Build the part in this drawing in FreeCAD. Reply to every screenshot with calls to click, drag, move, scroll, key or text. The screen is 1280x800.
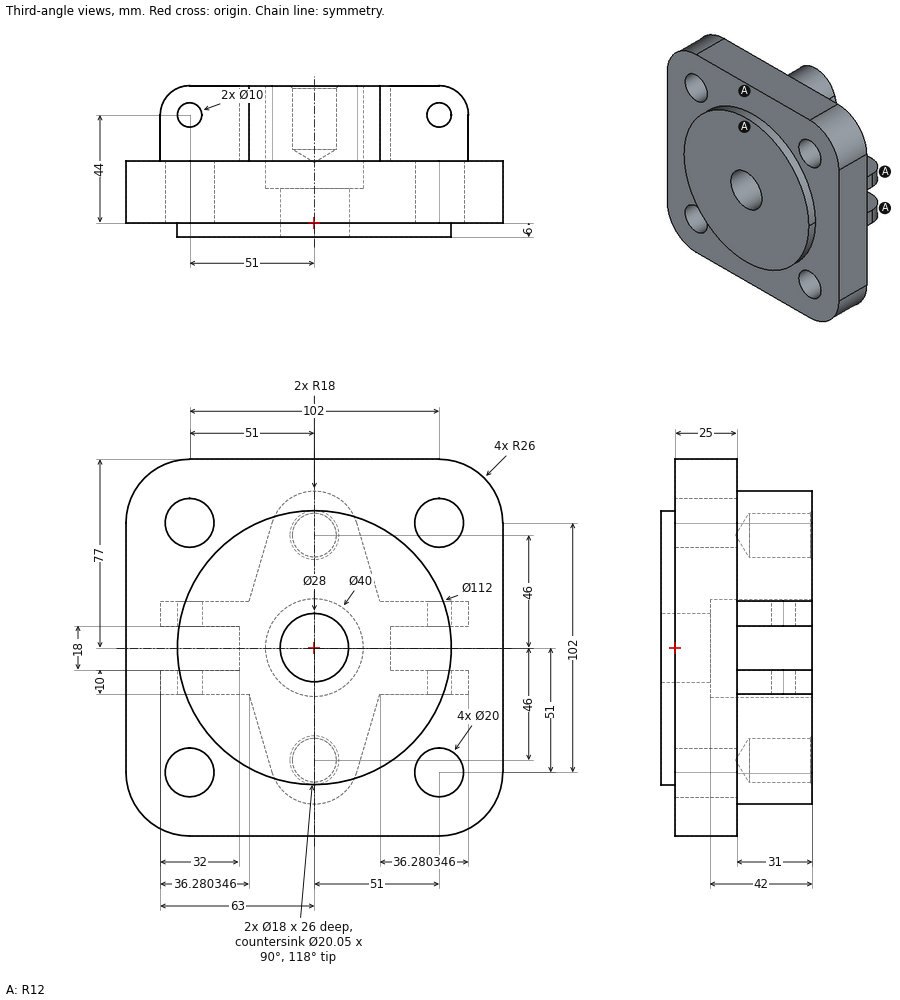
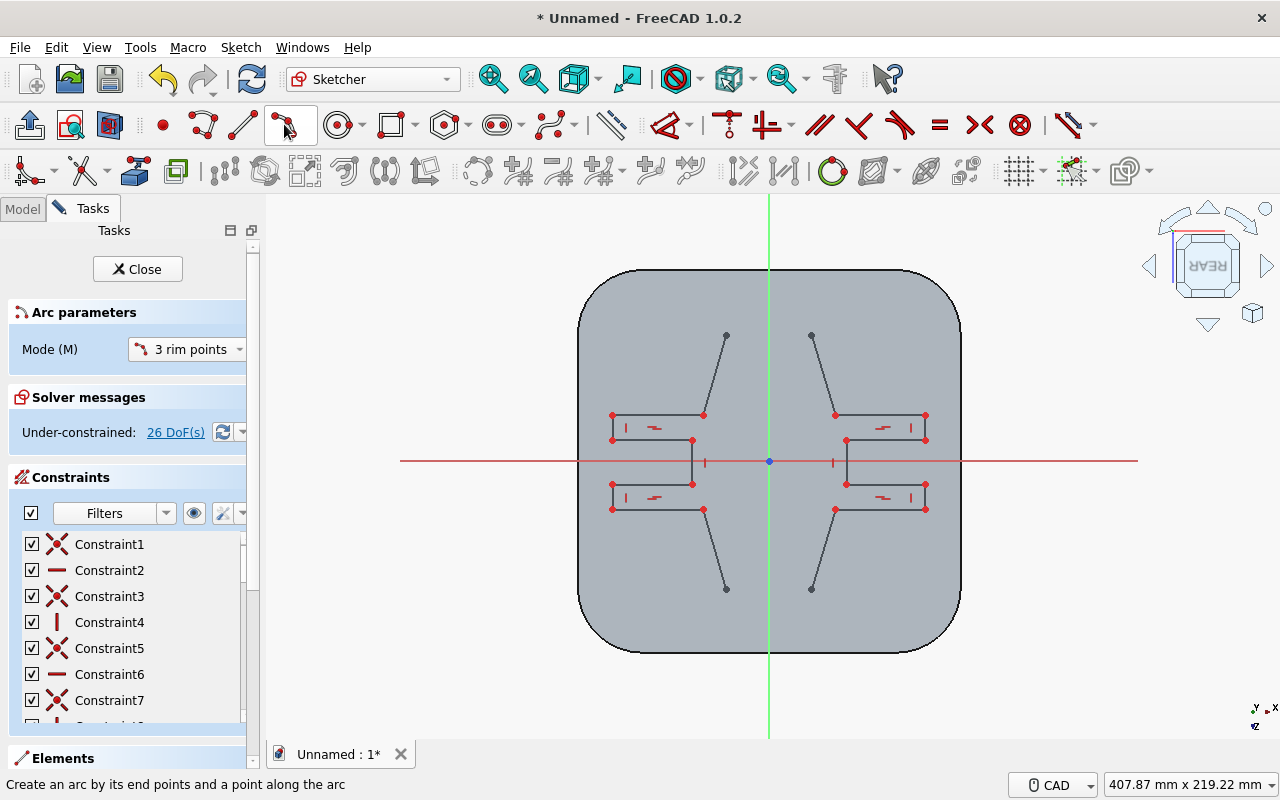
click(726, 590)
click(812, 590)
click(747, 615)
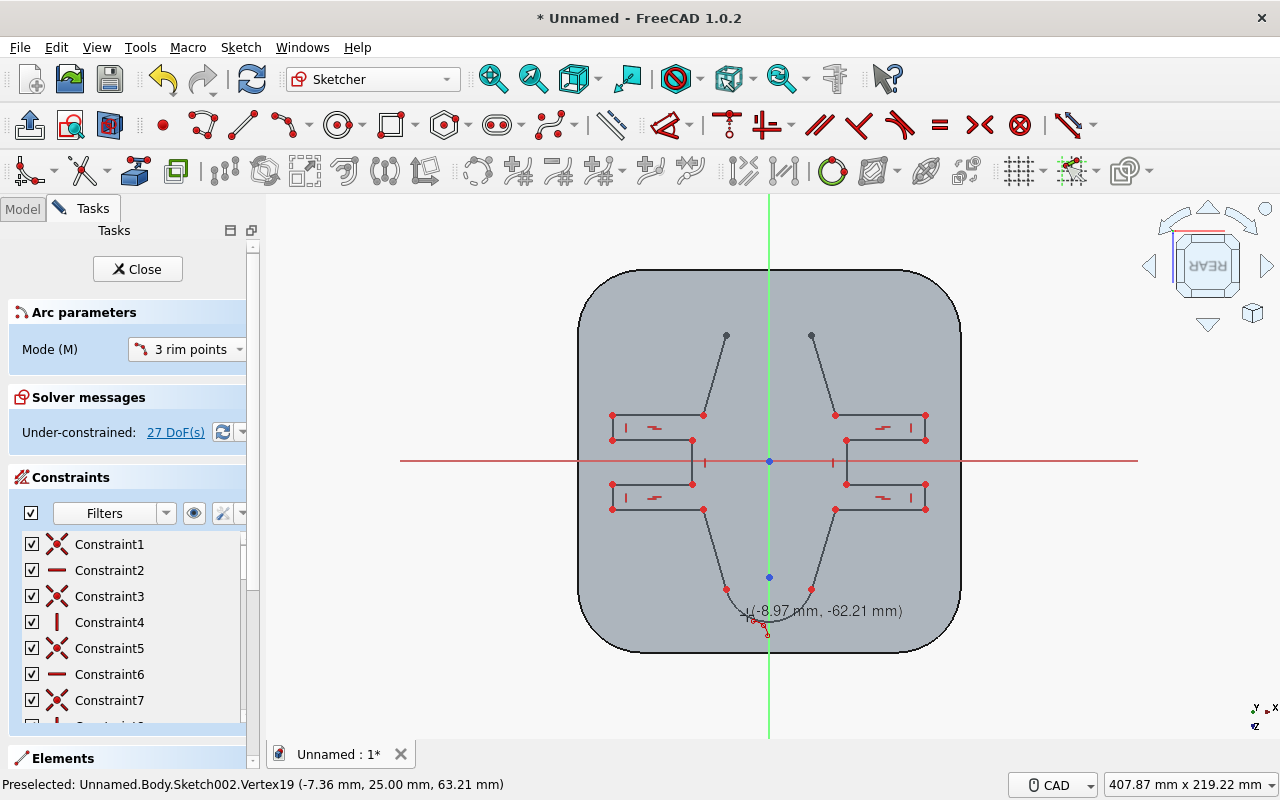
click(812, 335)
click(726, 335)
click(791, 308)
key(Escape)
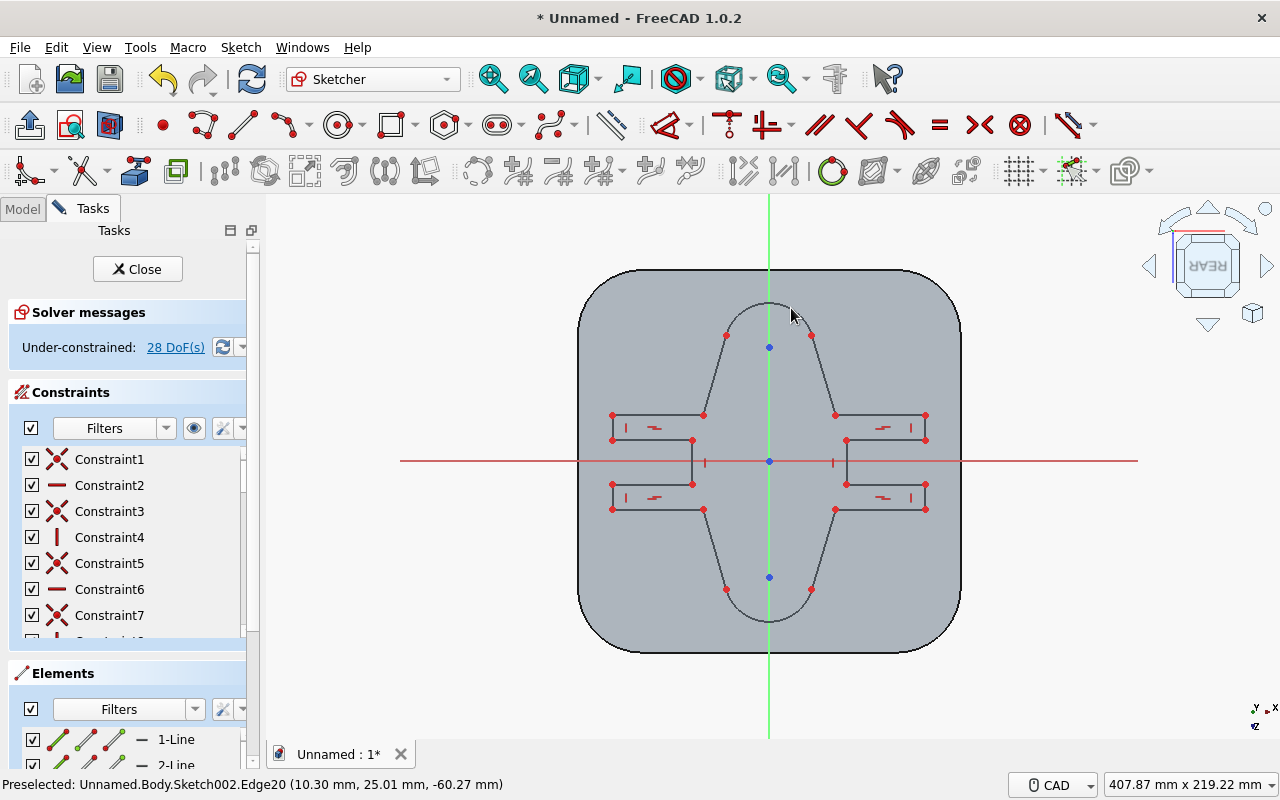
click(719, 359)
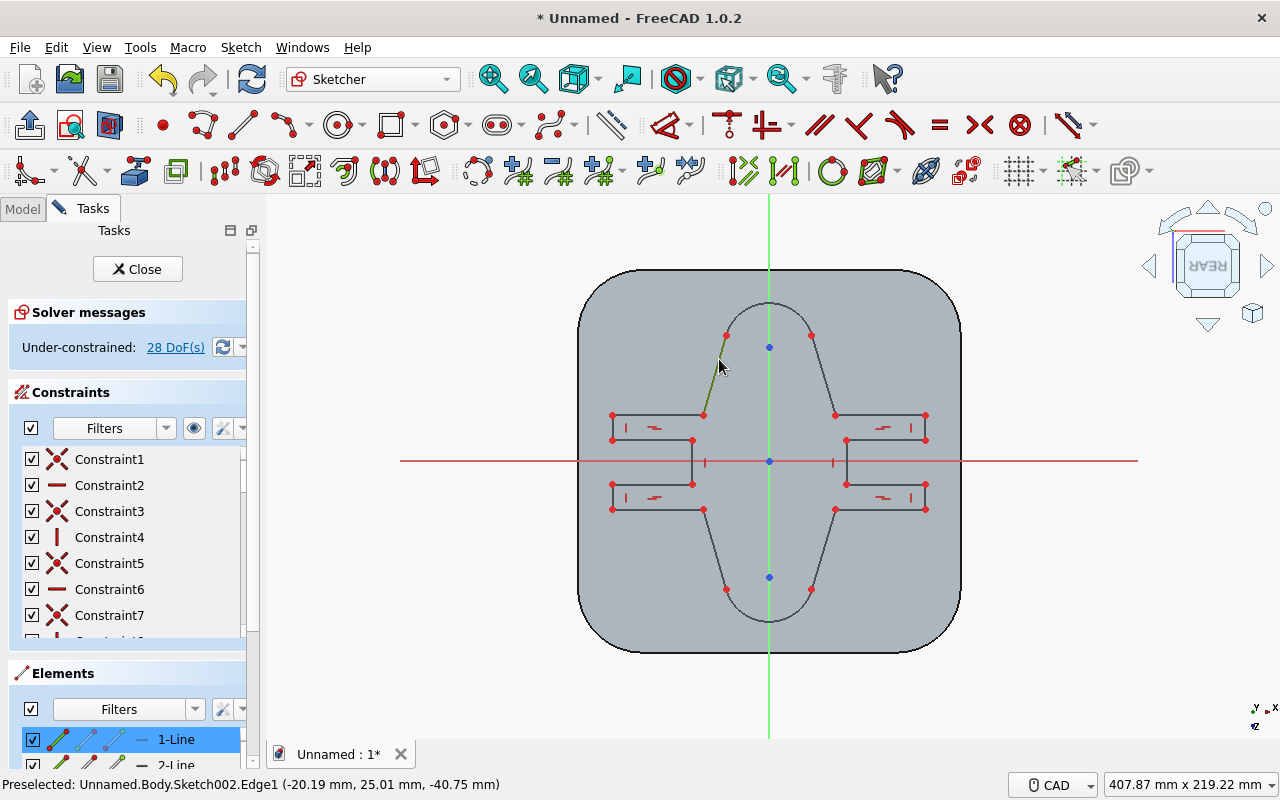
click(791, 309)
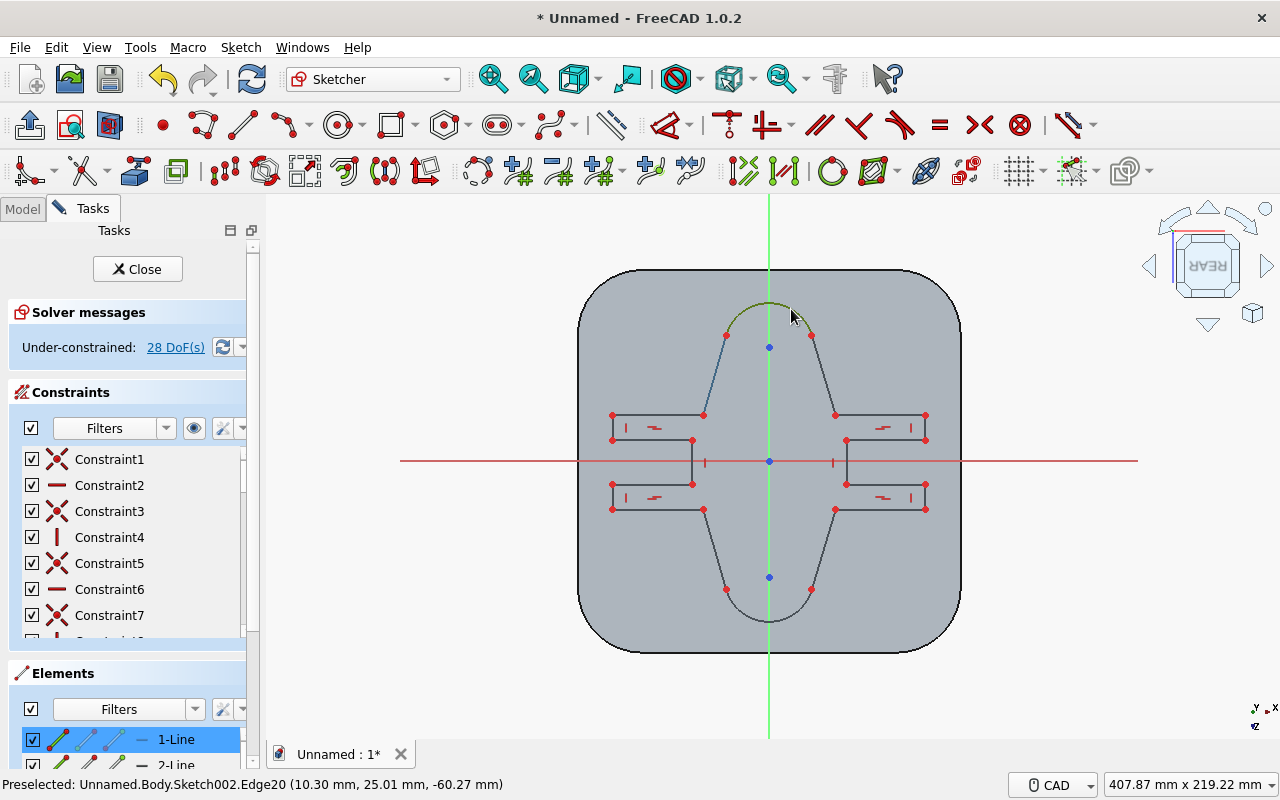
key(t)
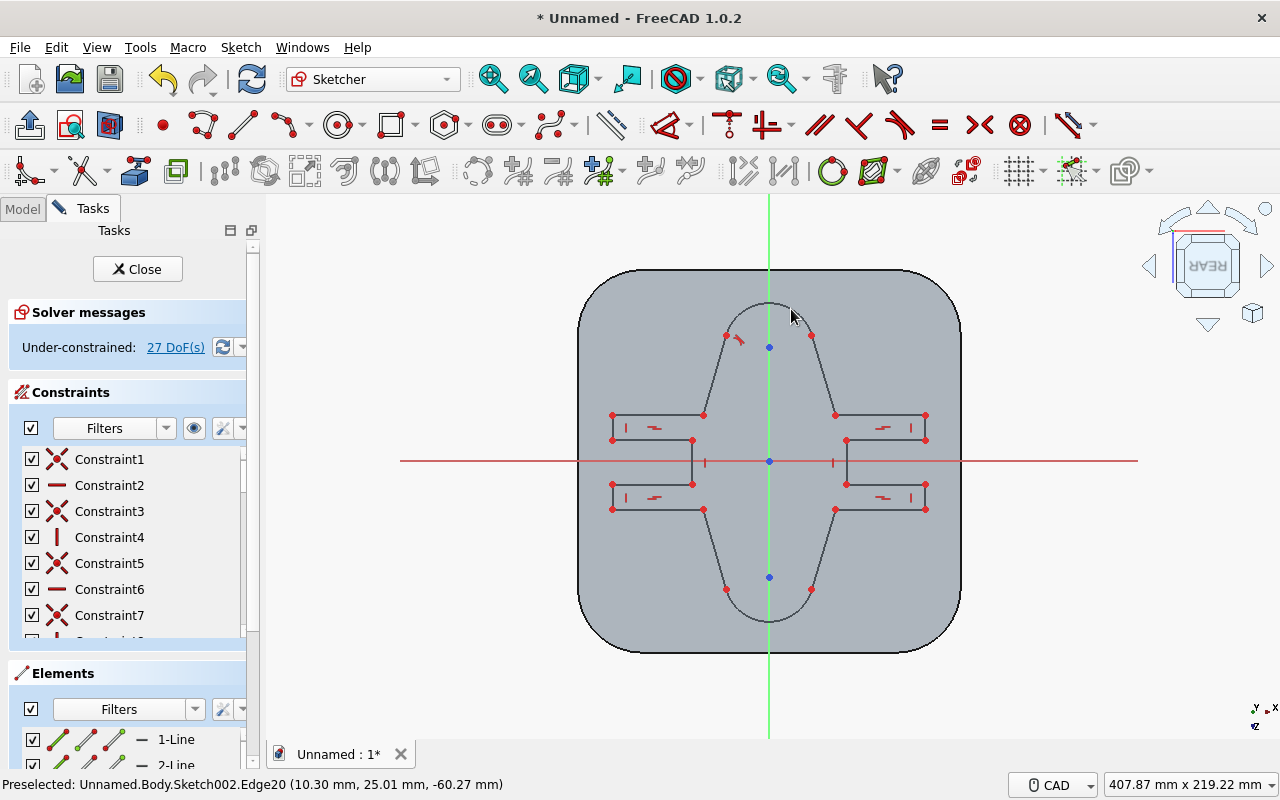
click(710, 534)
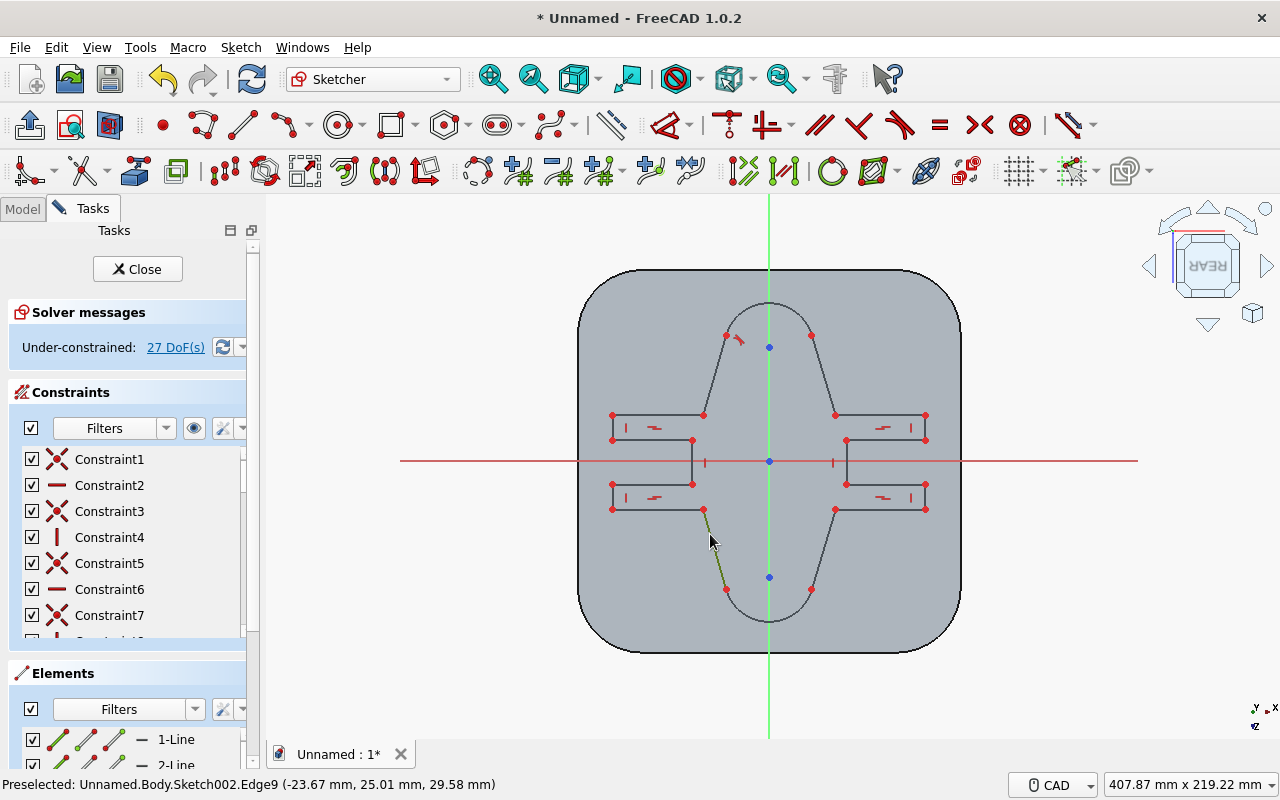
click(747, 616)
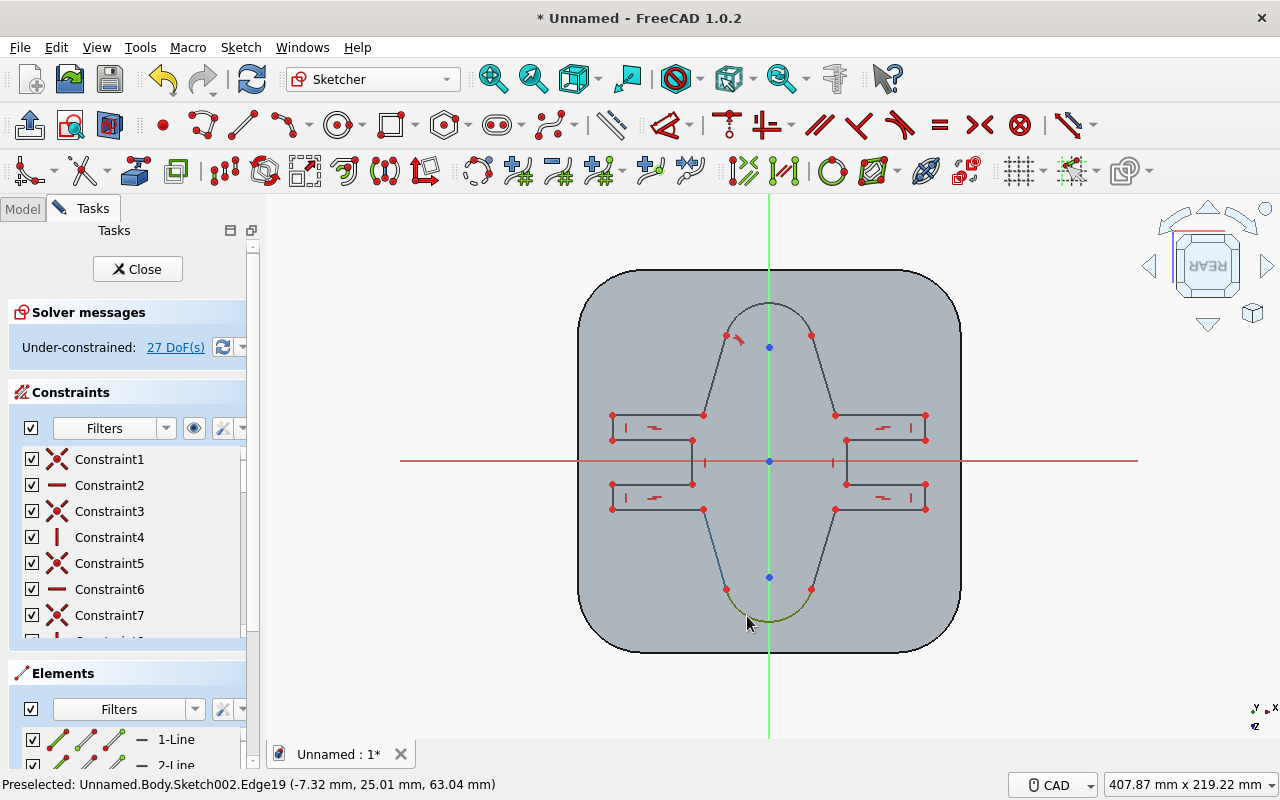
key(t)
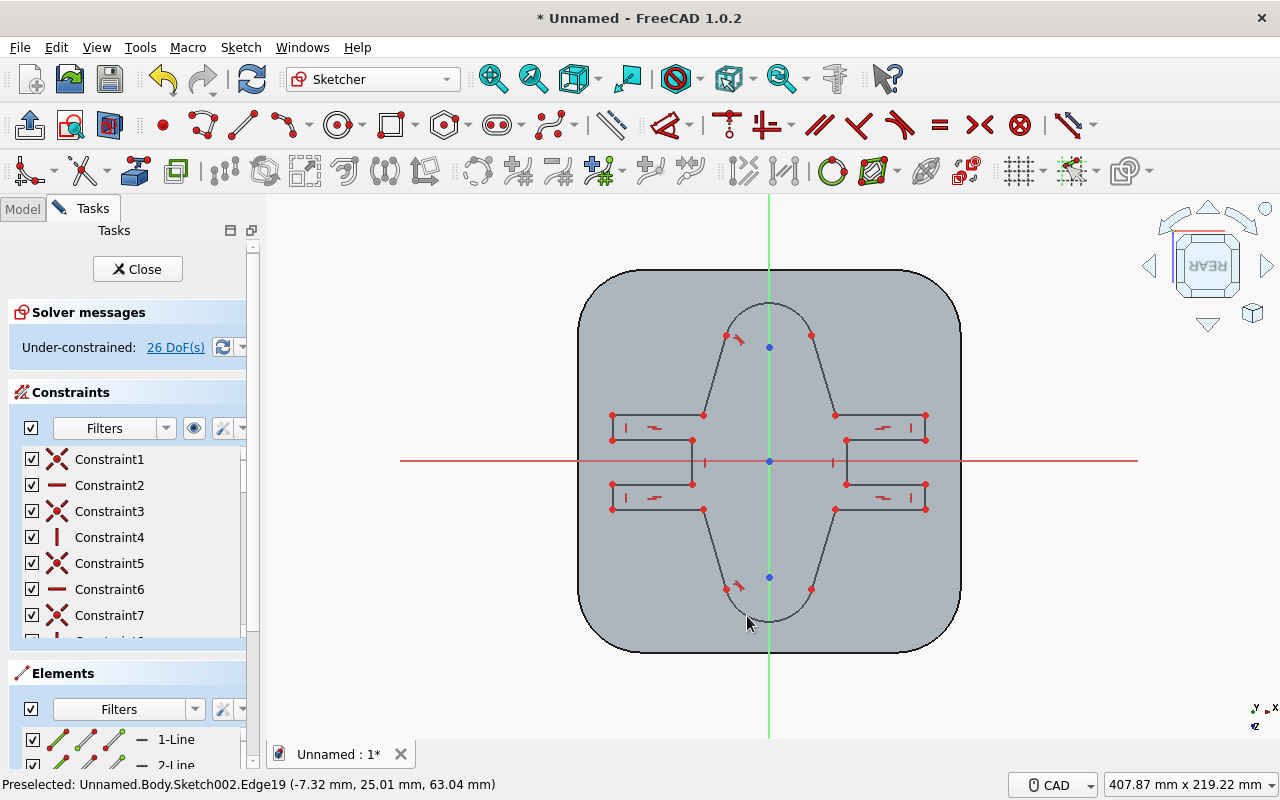
click(819, 566)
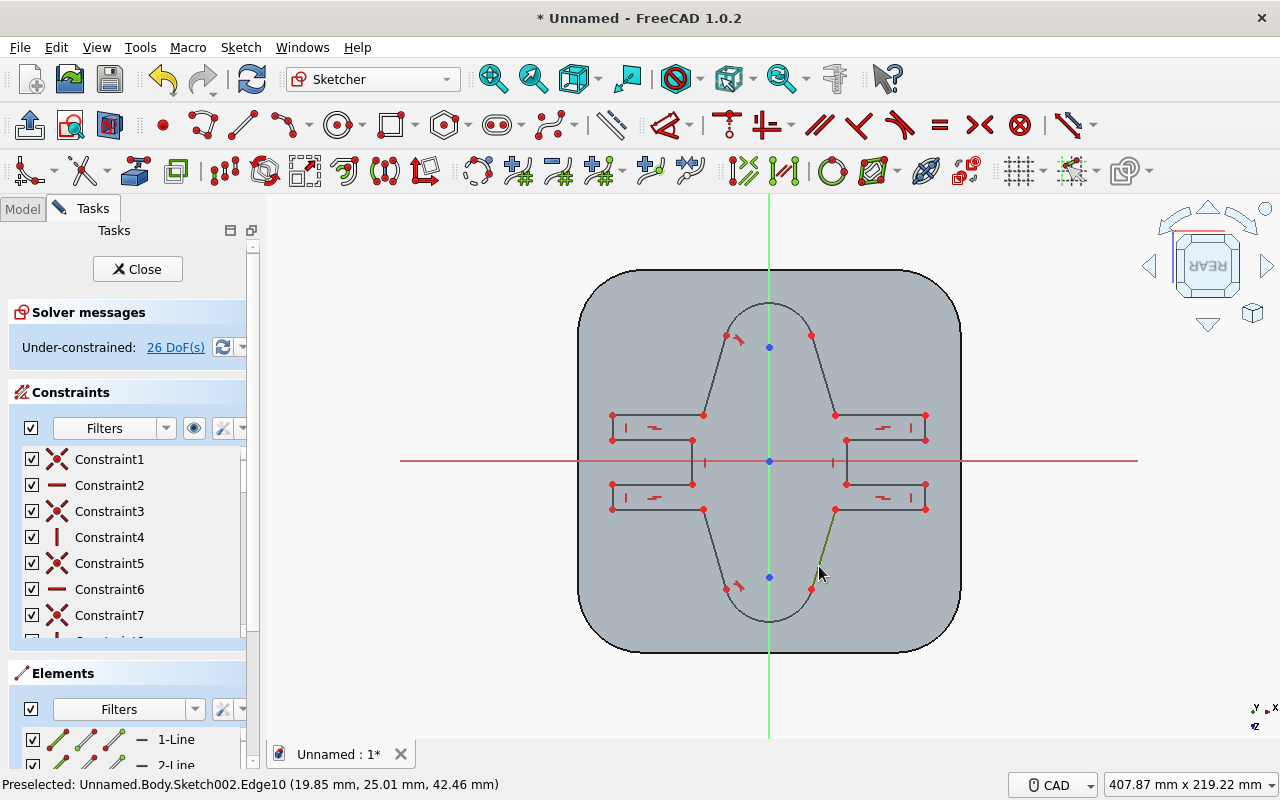
click(747, 616)